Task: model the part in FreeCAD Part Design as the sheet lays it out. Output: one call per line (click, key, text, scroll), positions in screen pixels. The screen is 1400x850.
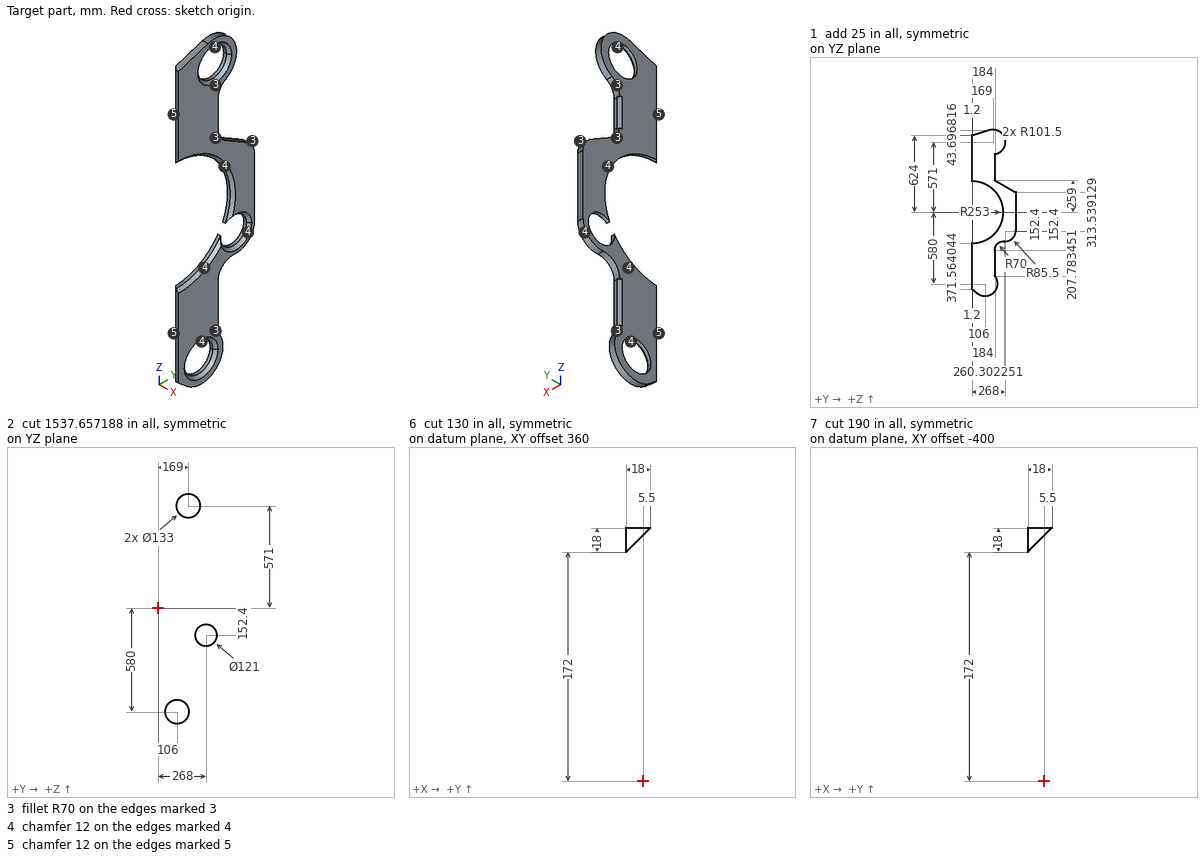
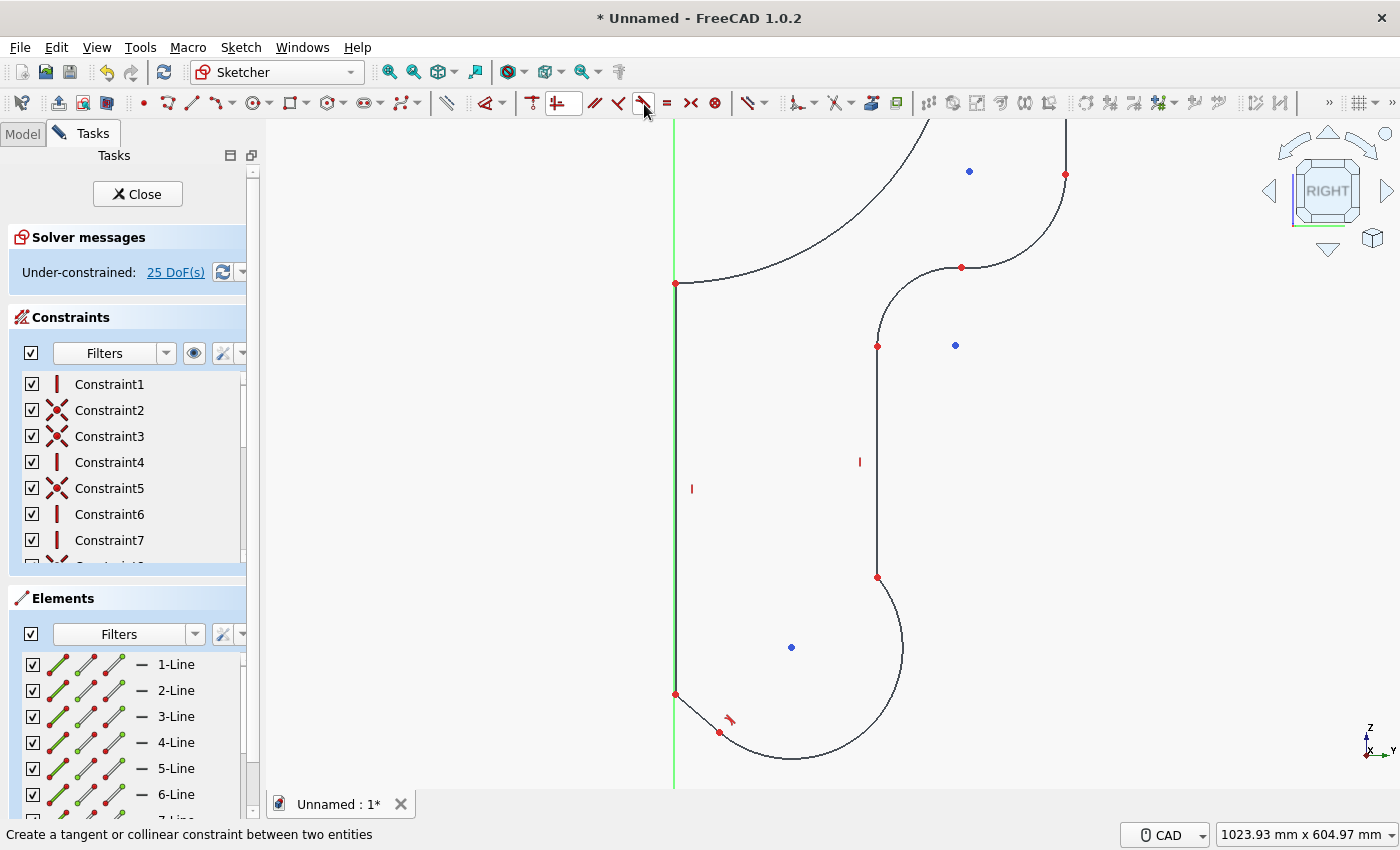
scroll(719, 651, down, 6)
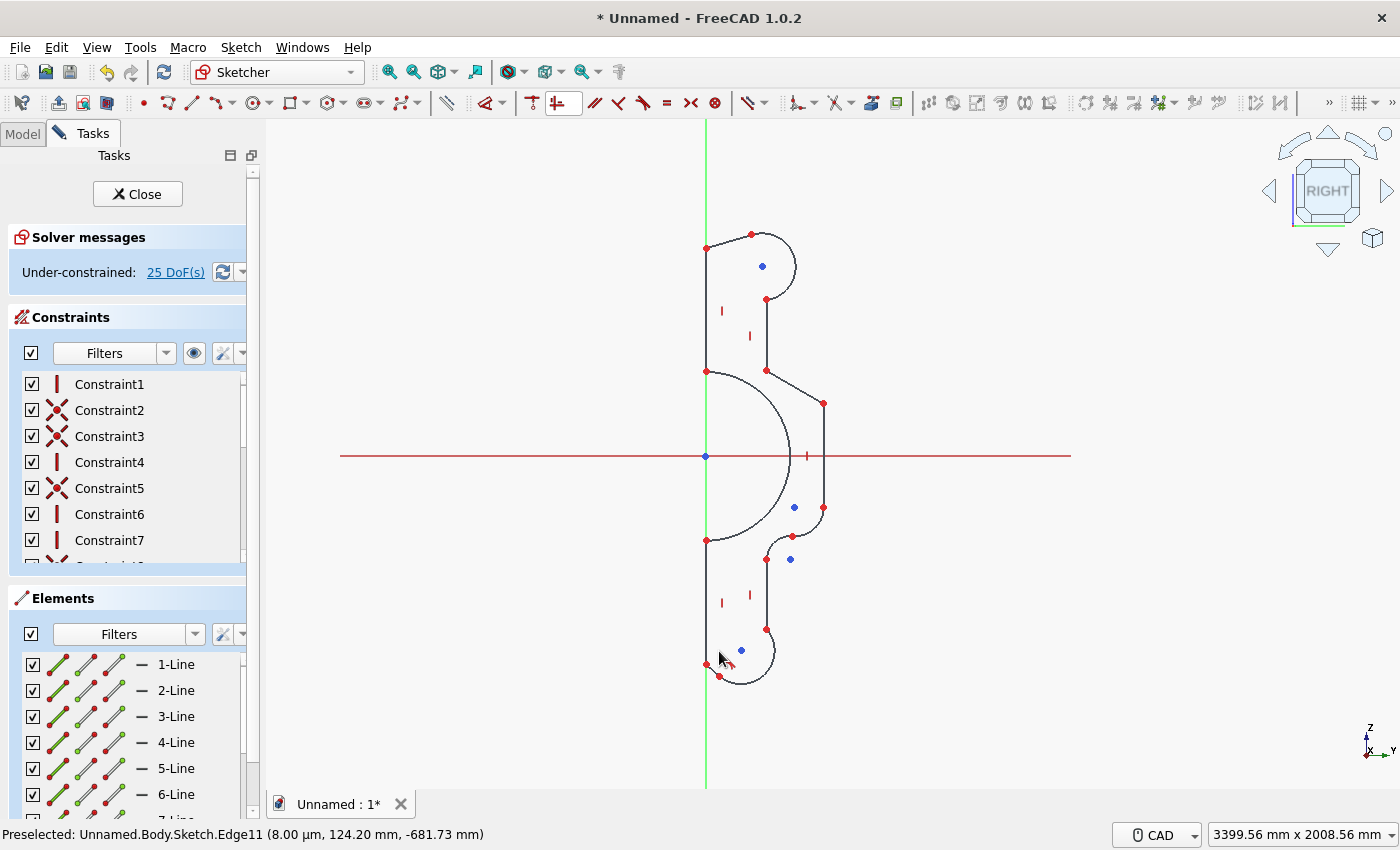
scroll(706, 456, up, 3)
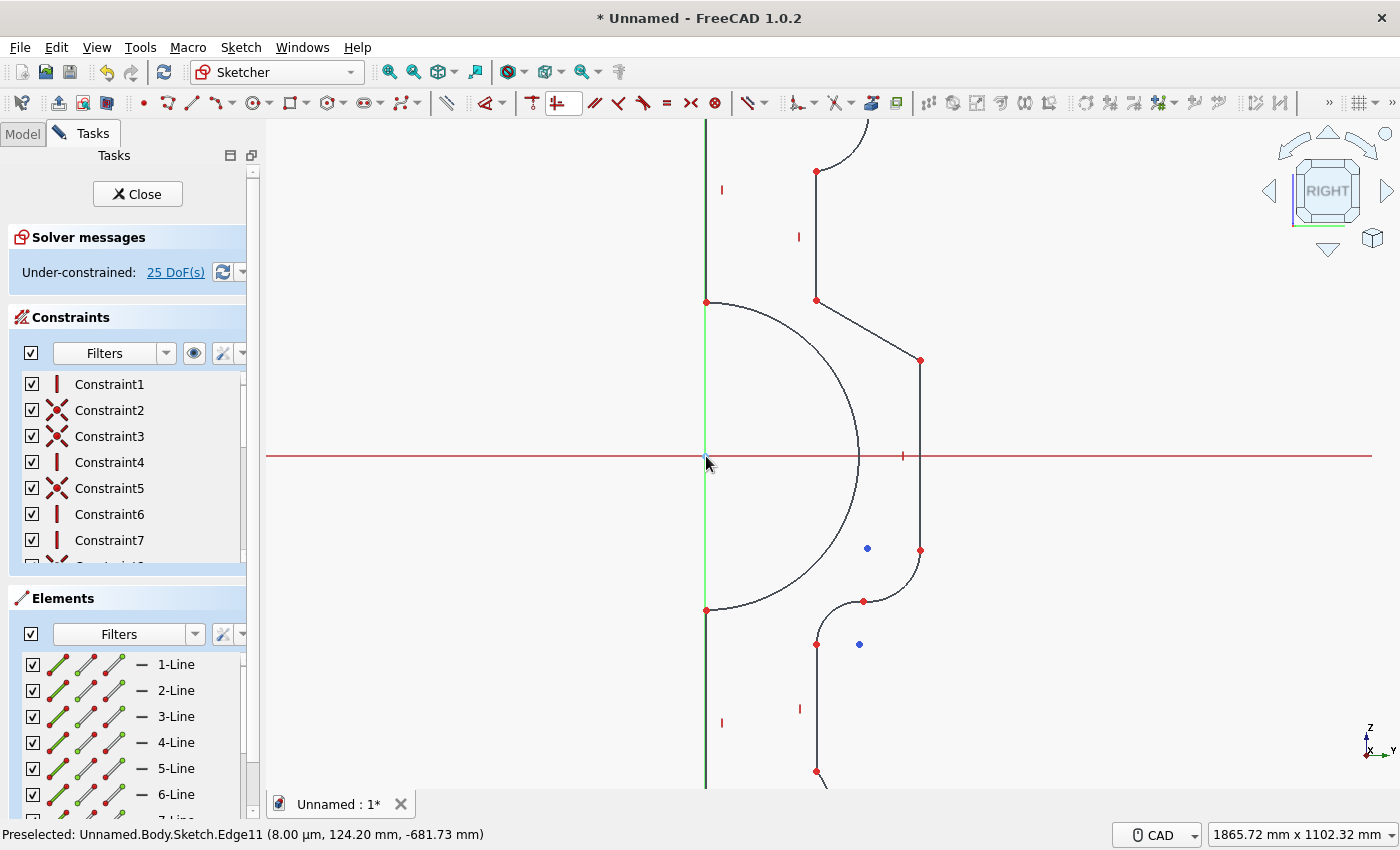
drag(695, 446, 715, 466)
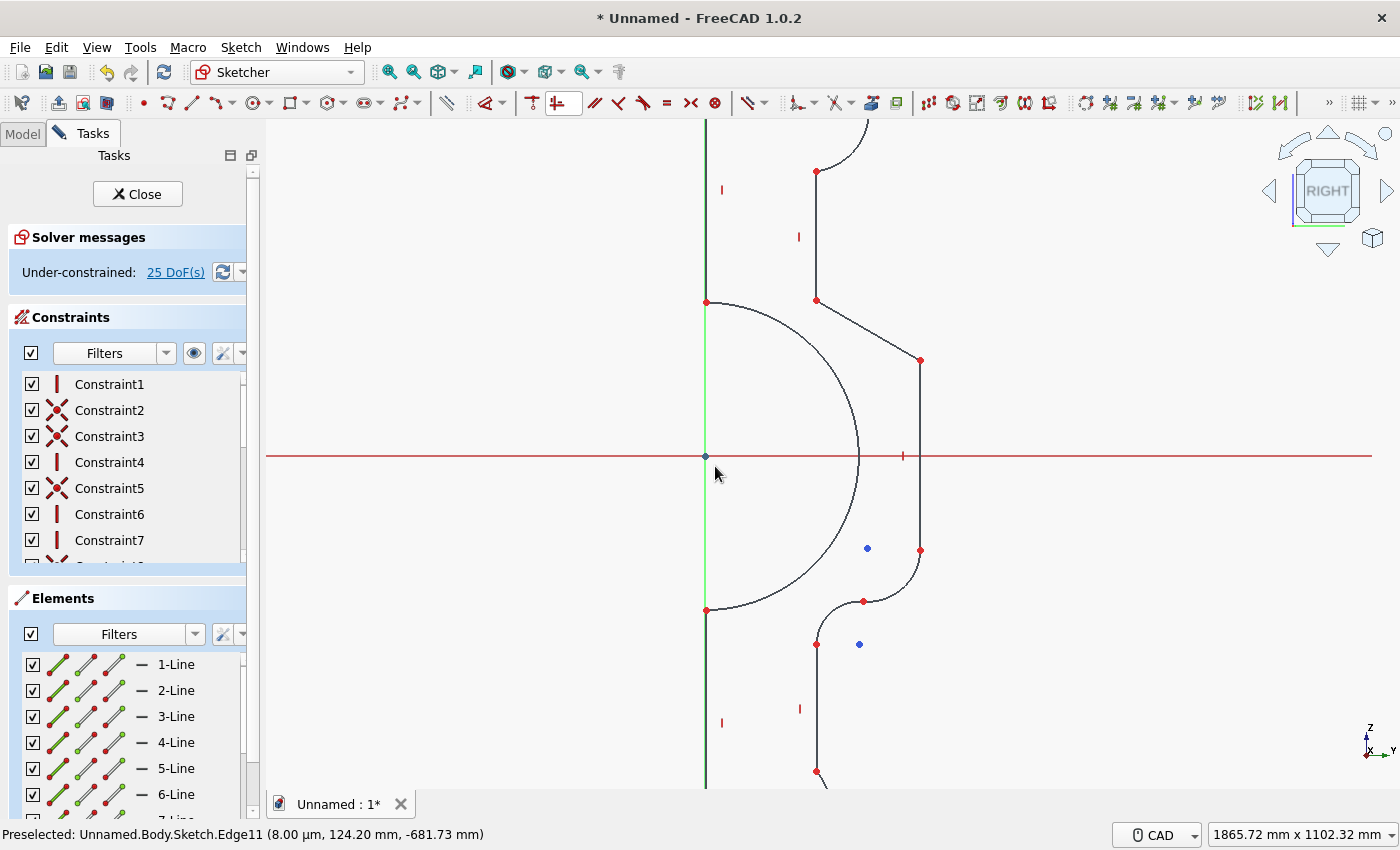
click(532, 104)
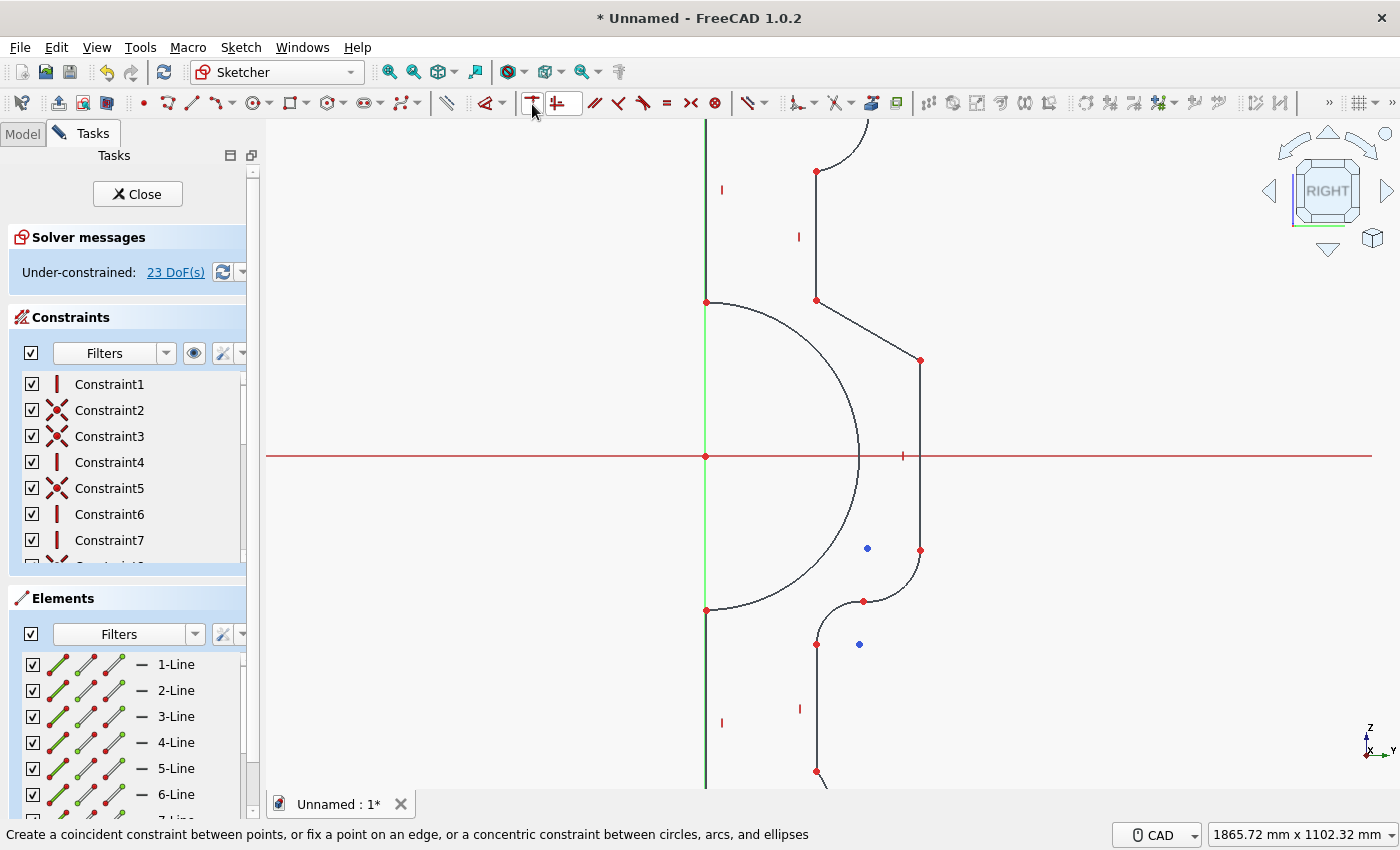
click(852, 153)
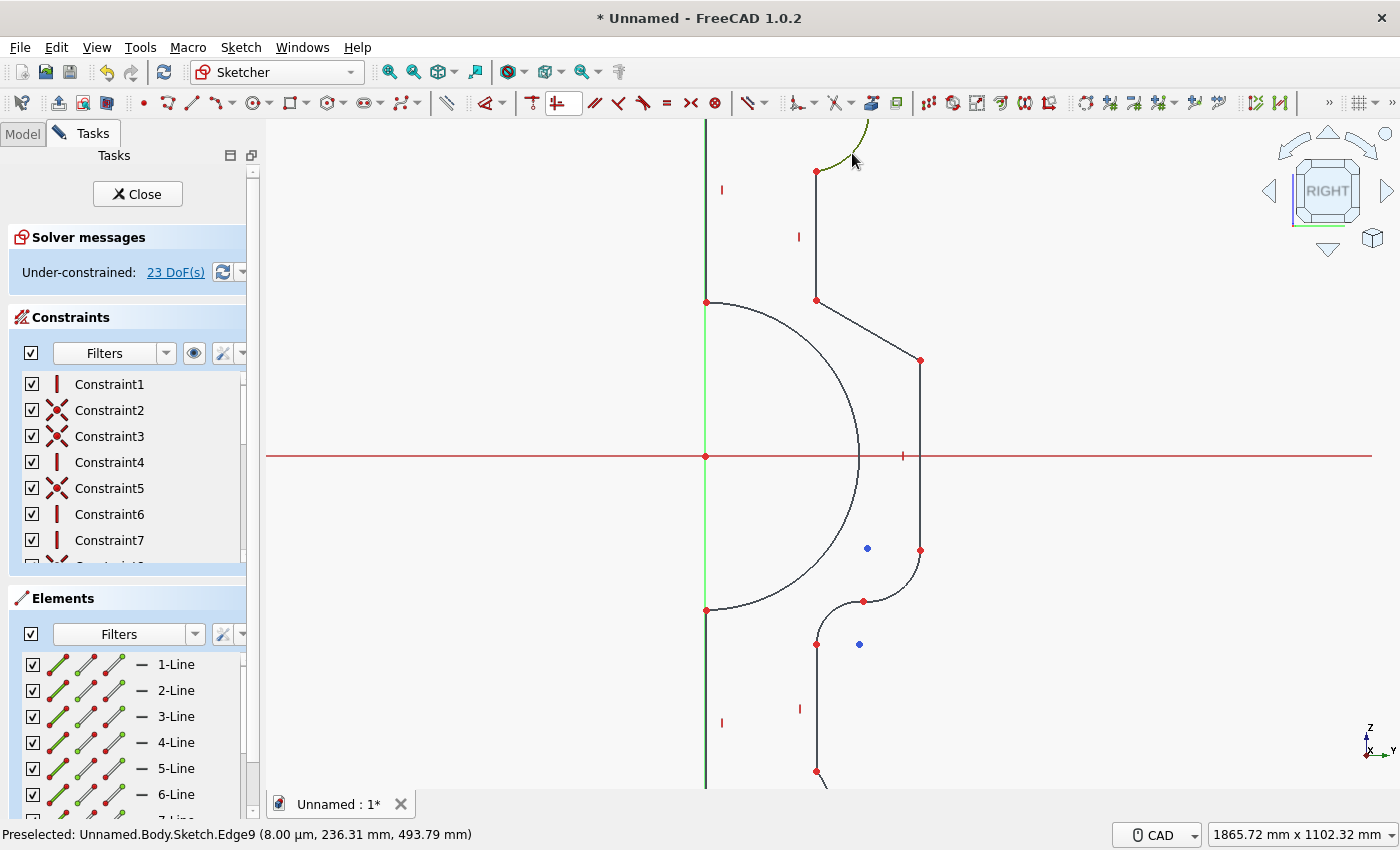
scroll(706, 455, down, 3)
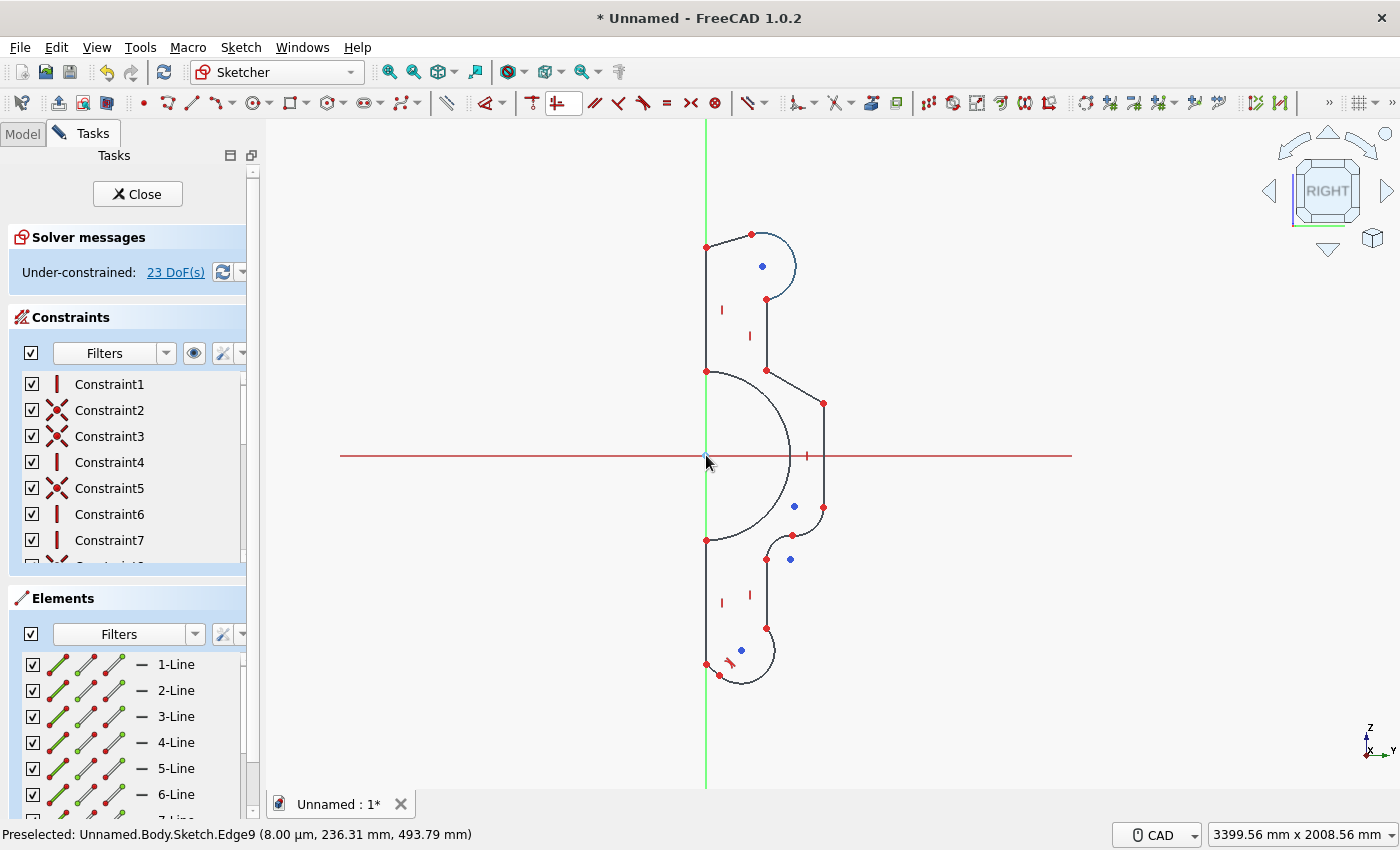
click(747, 683)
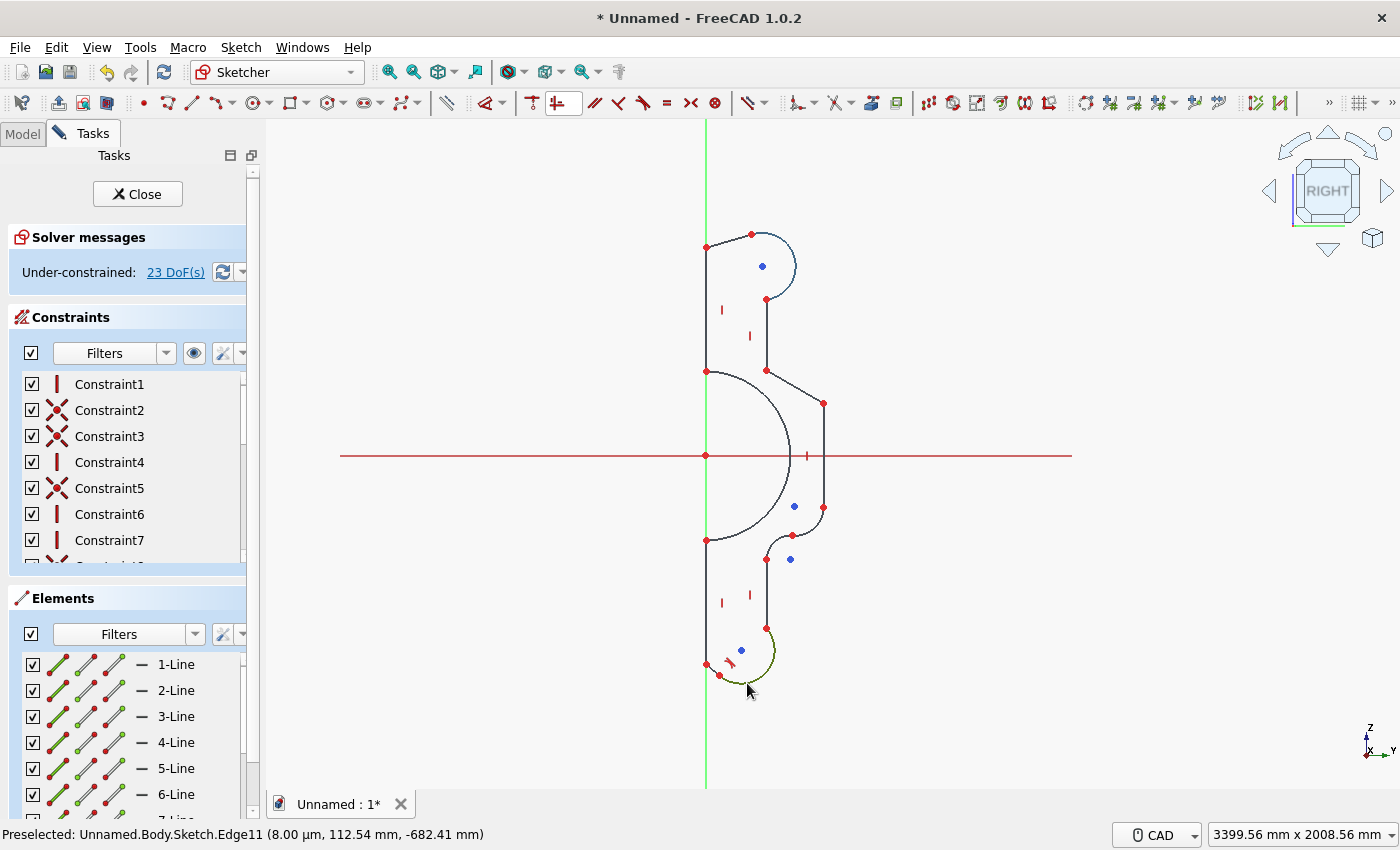
key(e)